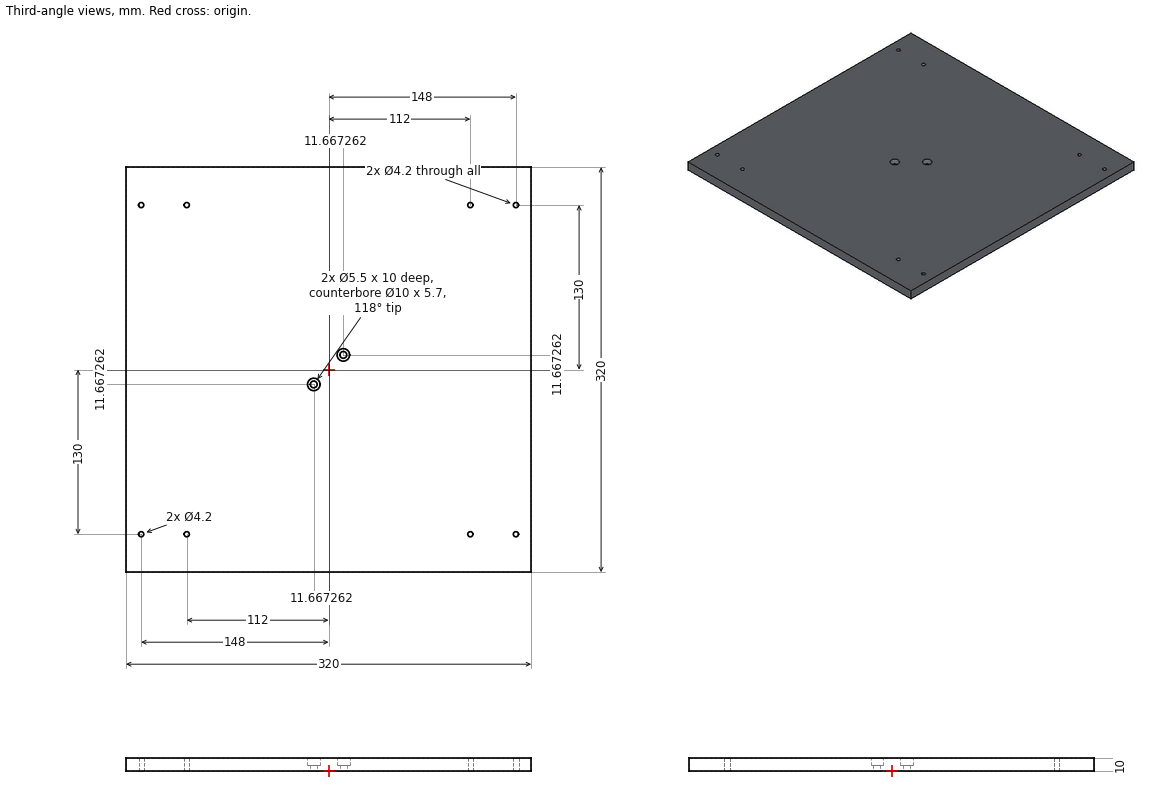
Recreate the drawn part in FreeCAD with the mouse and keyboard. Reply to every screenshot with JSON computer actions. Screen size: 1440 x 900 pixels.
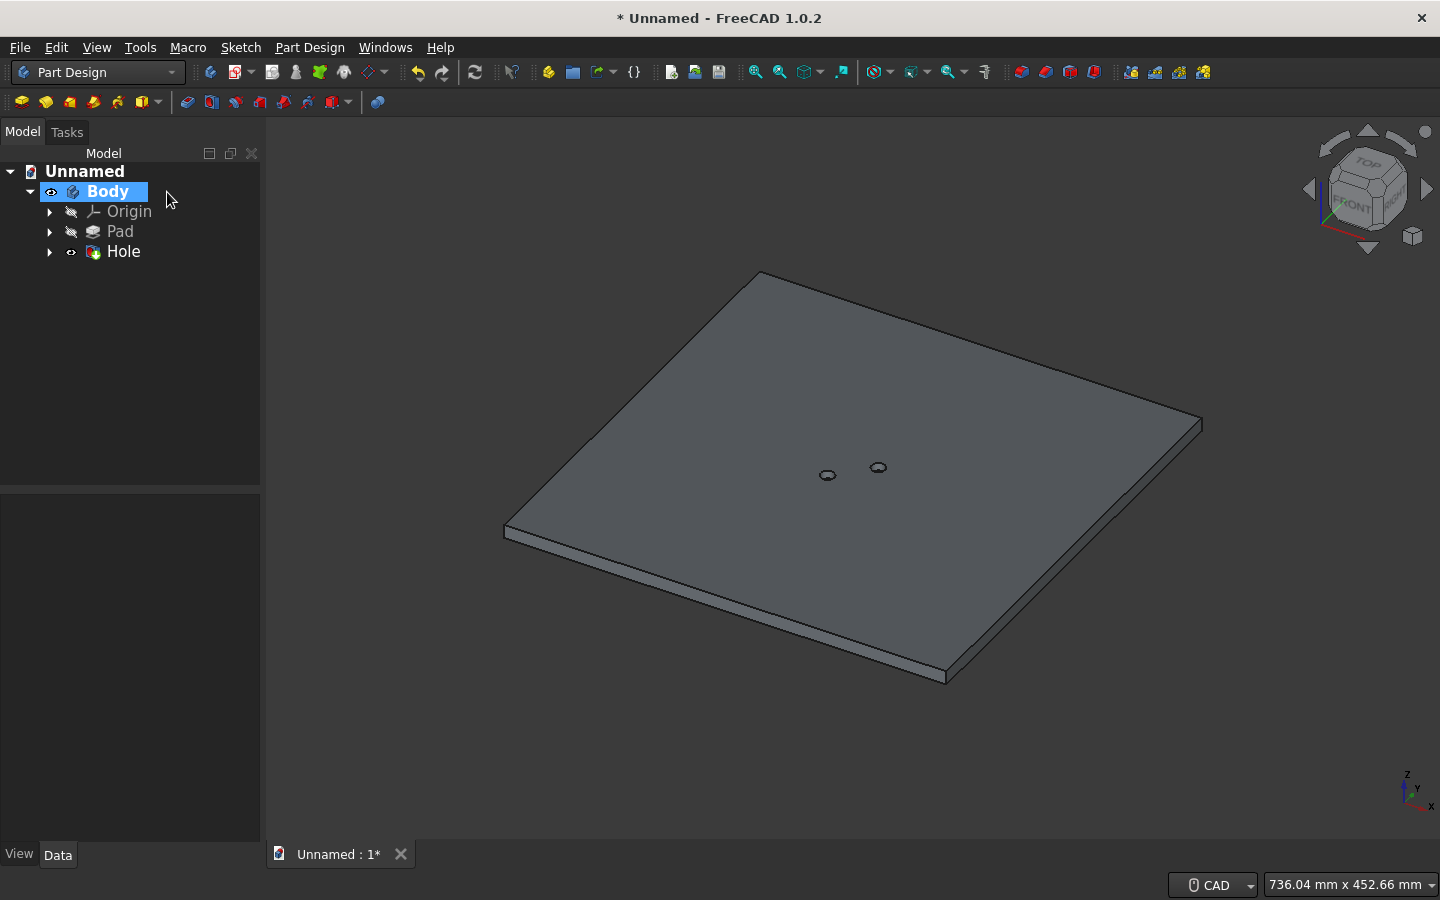
{"action": "left_click", "coordinate": [236, 72]}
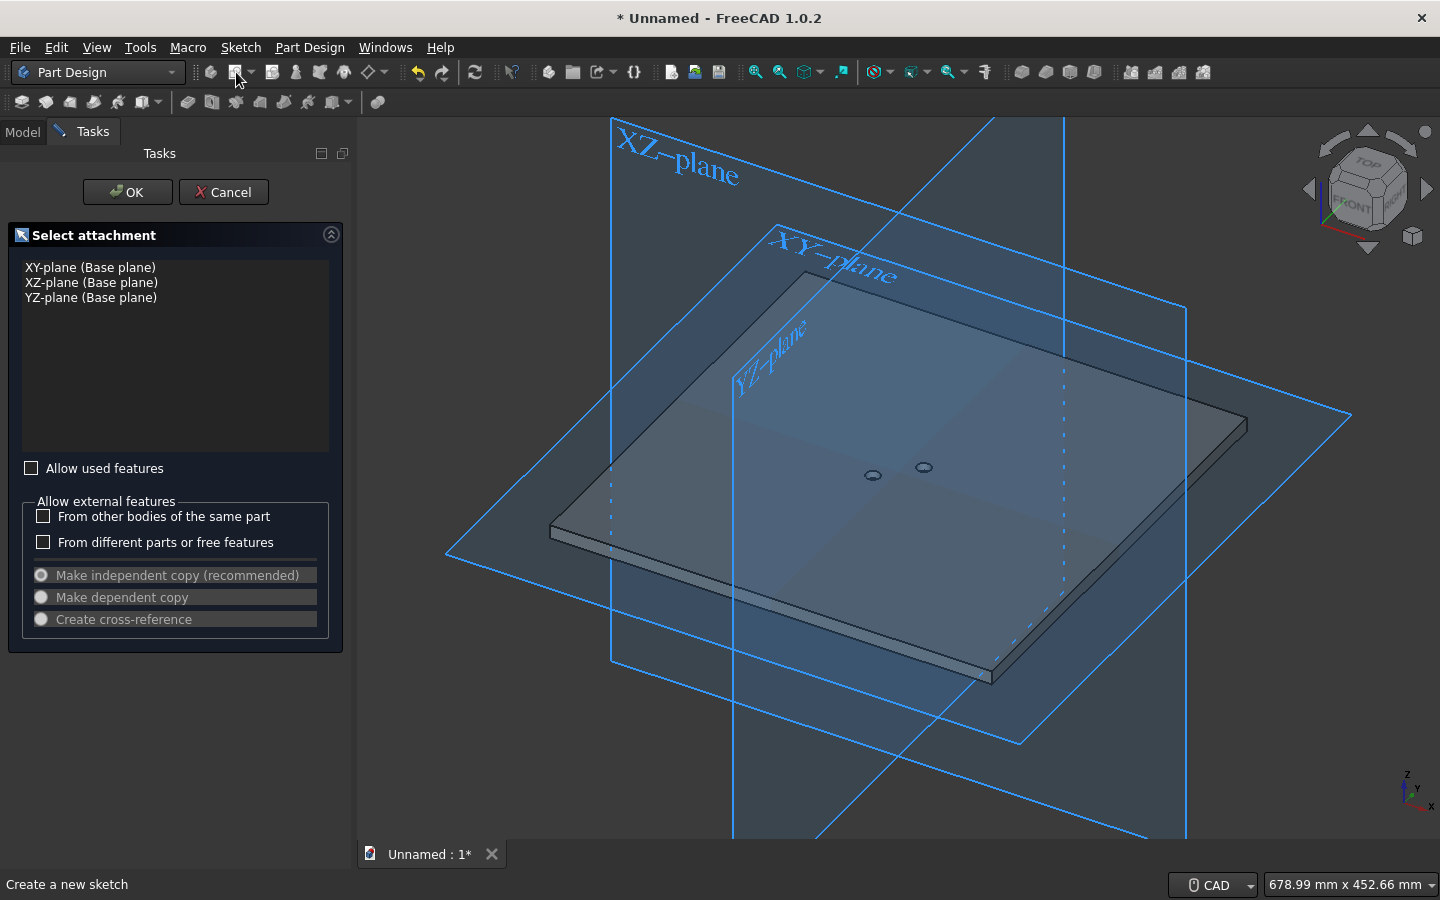
{"action": "left_click", "coordinate": [82, 268]}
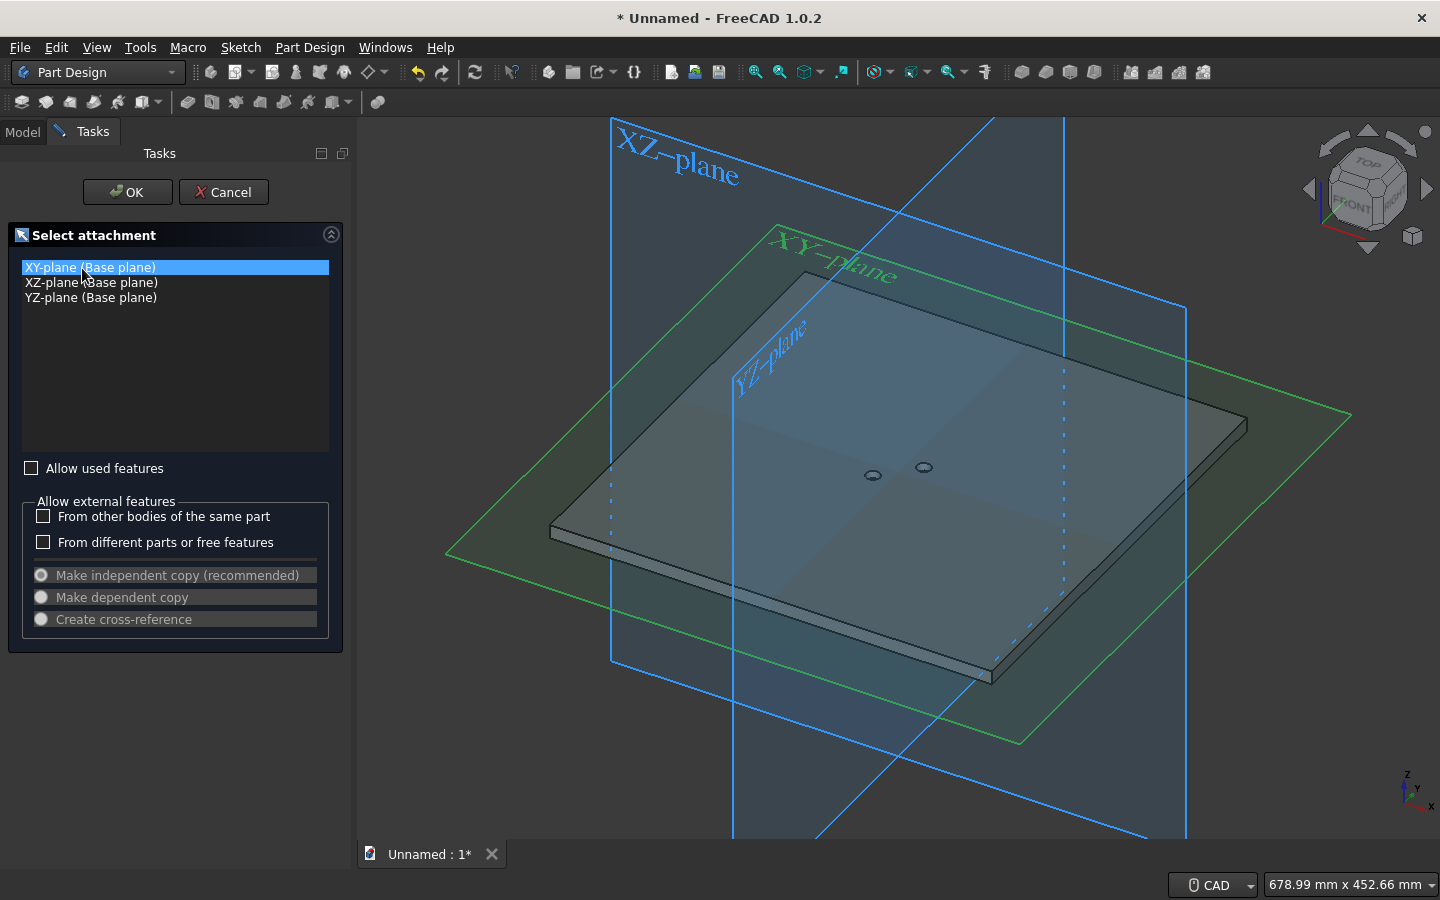
{"action": "left_click", "coordinate": [128, 192]}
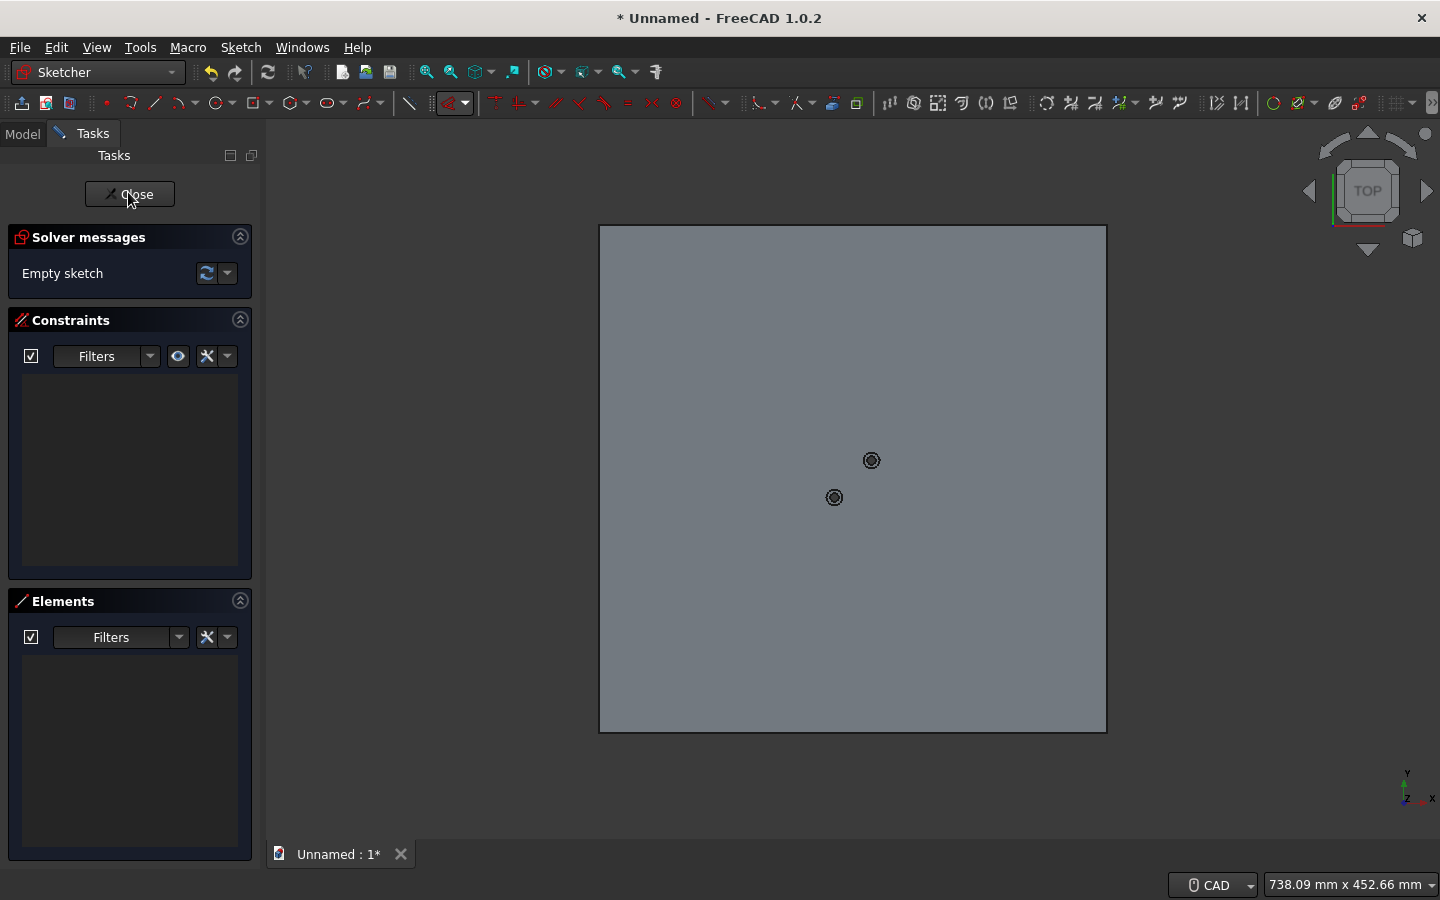
{"action": "left_click", "coordinate": [70, 104]}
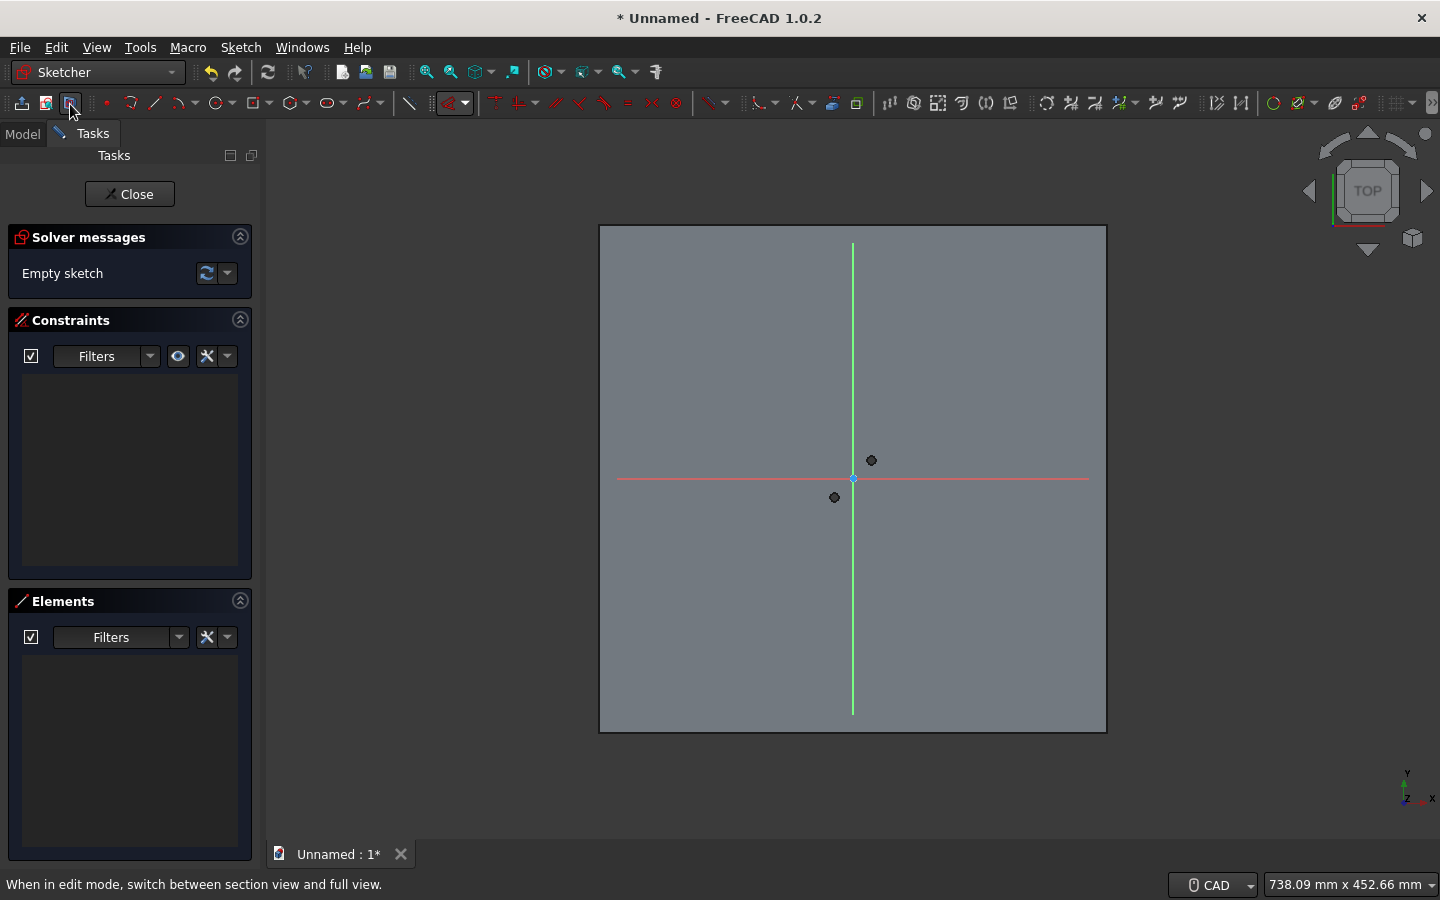
{"action": "scroll", "coordinate": [1087, 252], "scroll_direction": "up", "scroll_amount": 12}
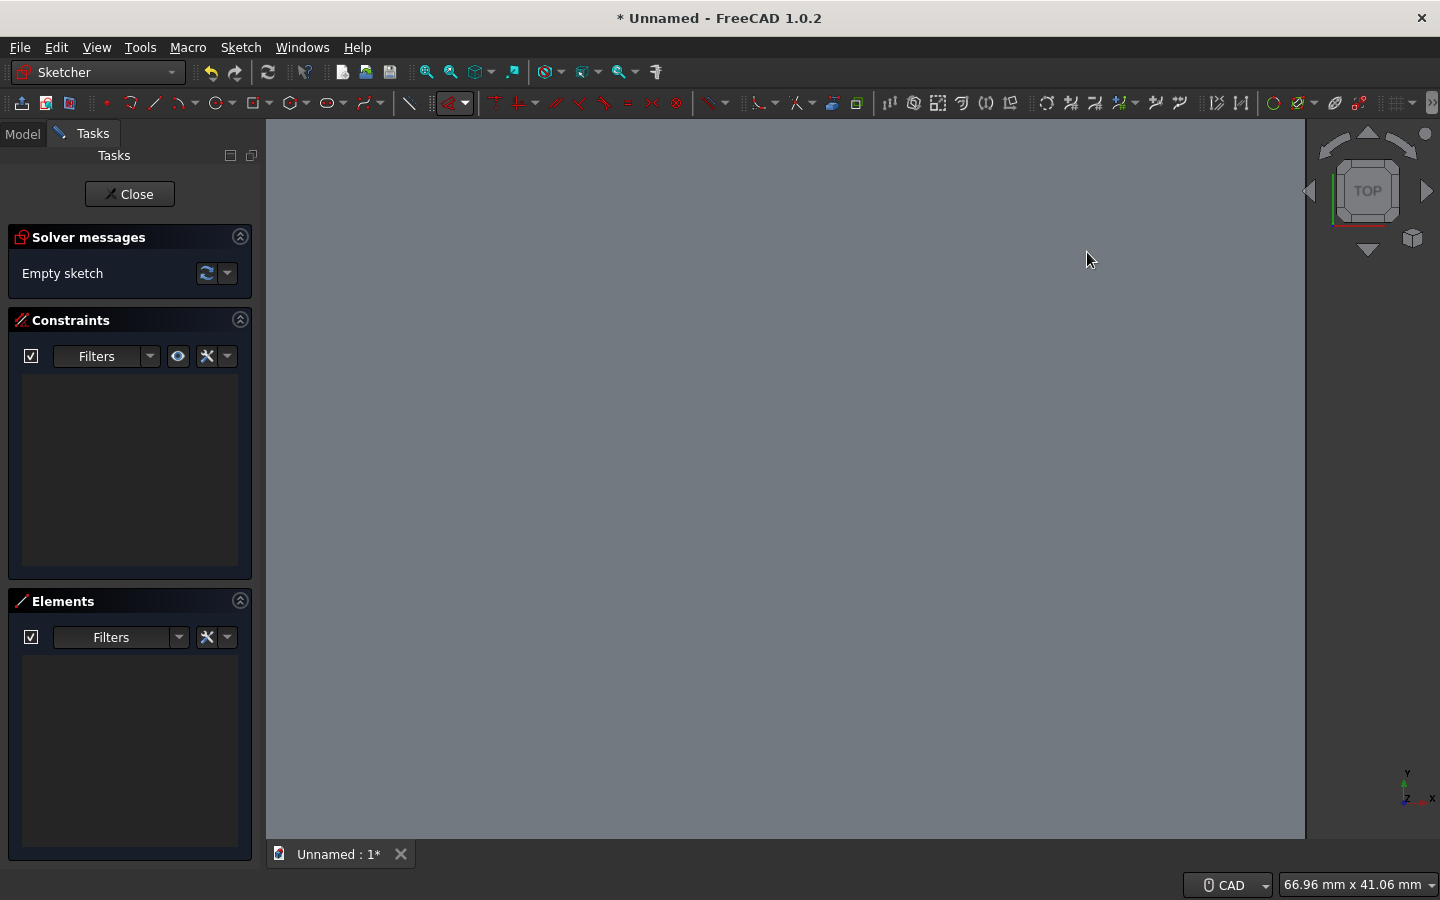
{"action": "left_click", "coordinate": [216, 104]}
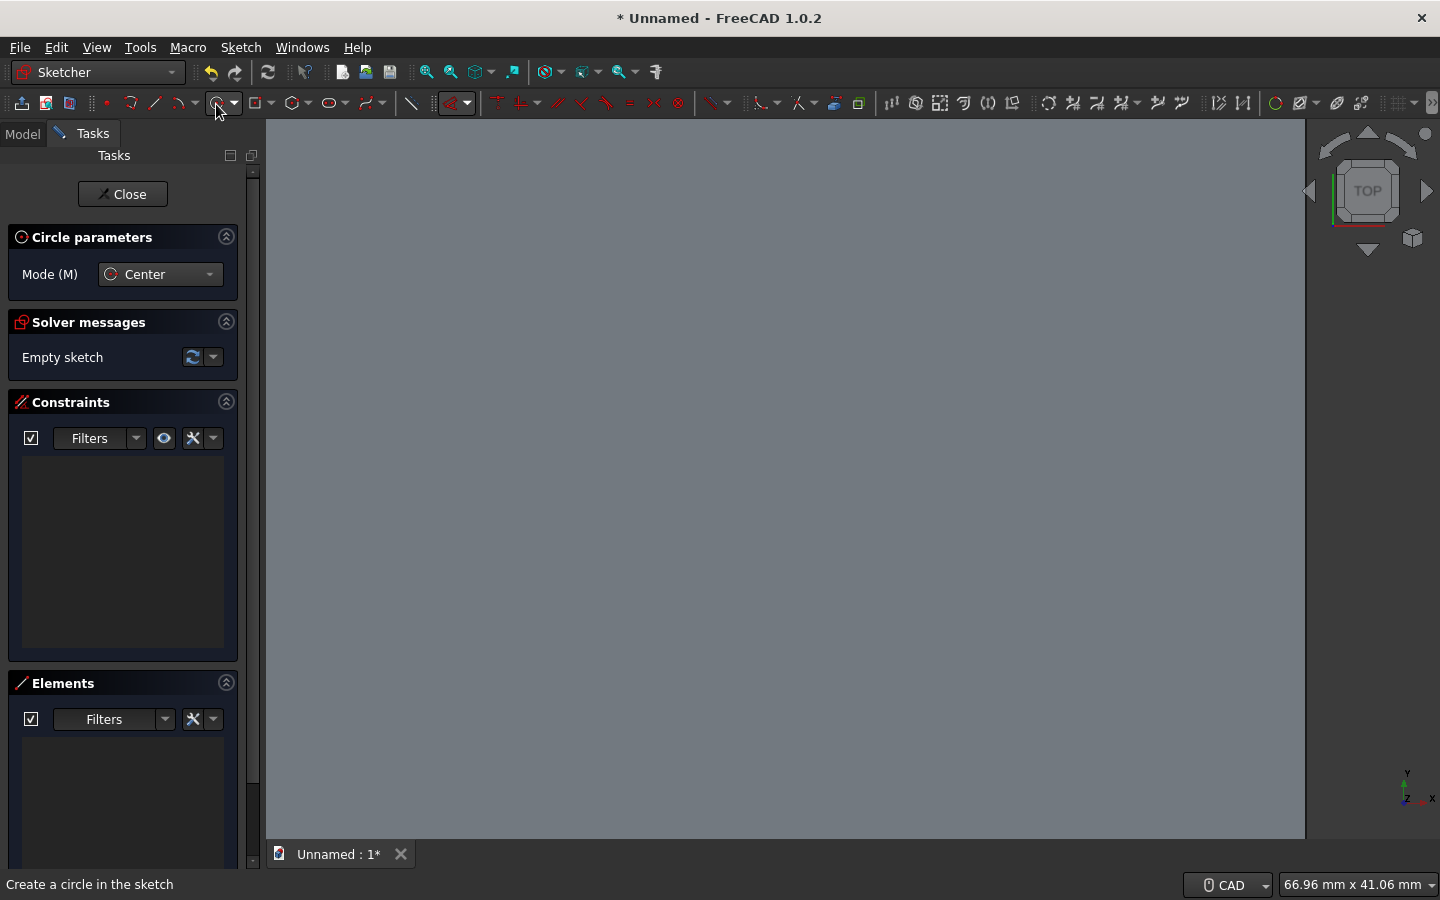
{"action": "left_click", "coordinate": [1096, 473]}
{"action": "mouse_move", "coordinate": [1122, 447]}